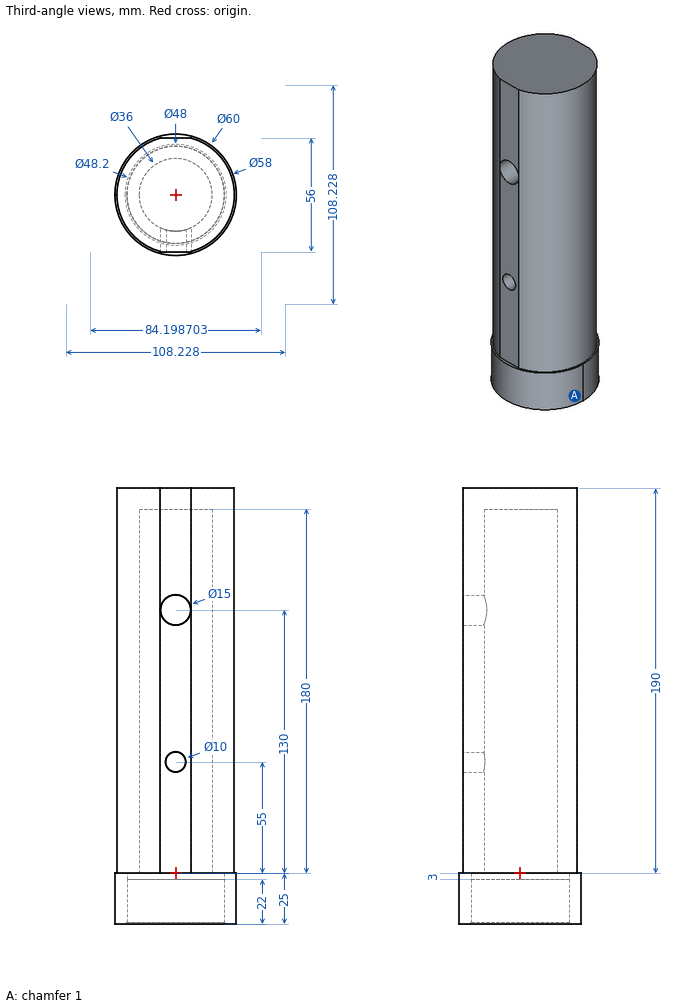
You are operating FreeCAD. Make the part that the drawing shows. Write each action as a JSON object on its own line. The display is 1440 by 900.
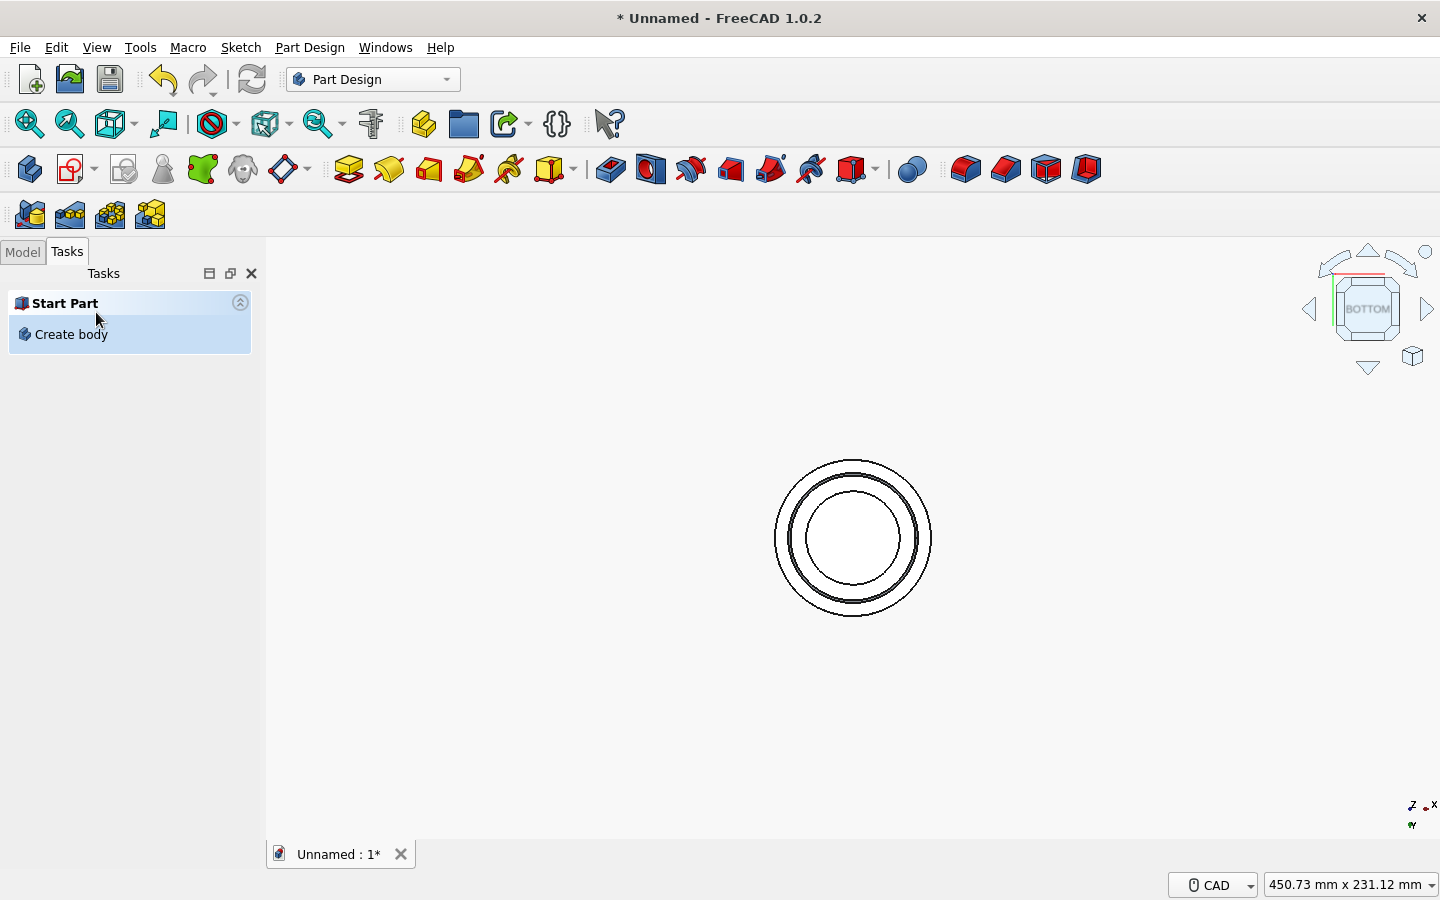
{"action": "key", "text": "0"}